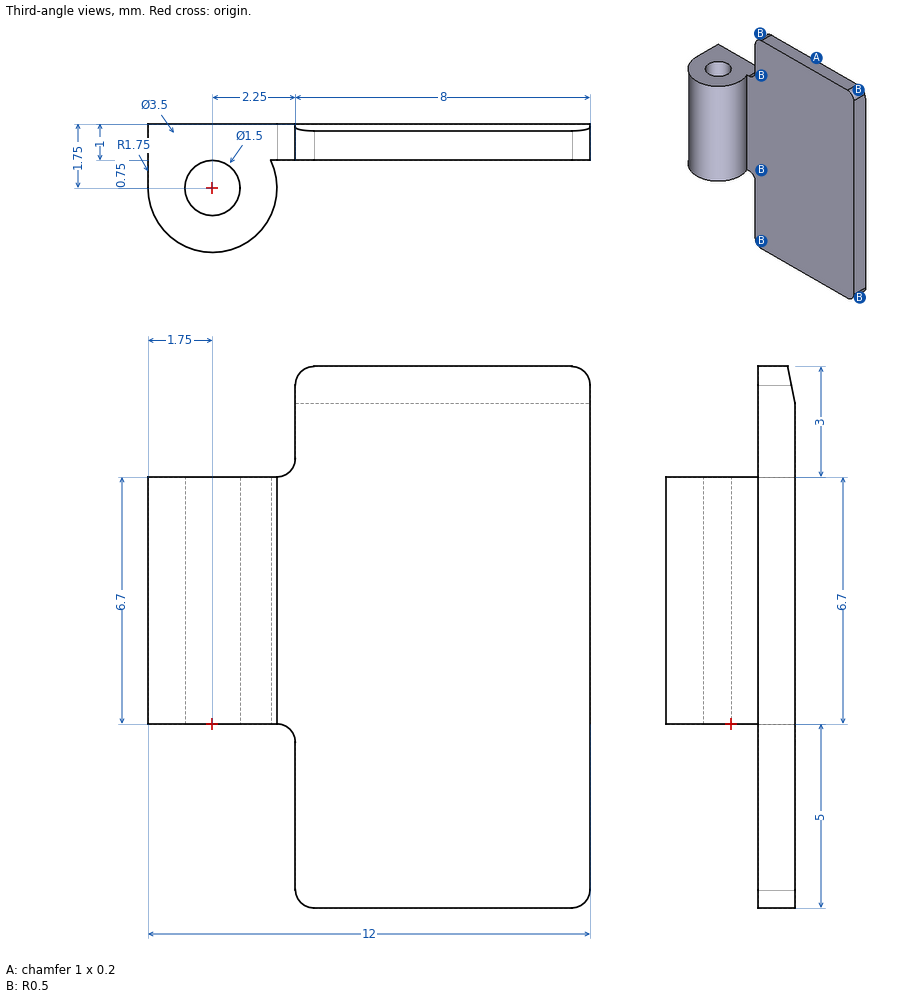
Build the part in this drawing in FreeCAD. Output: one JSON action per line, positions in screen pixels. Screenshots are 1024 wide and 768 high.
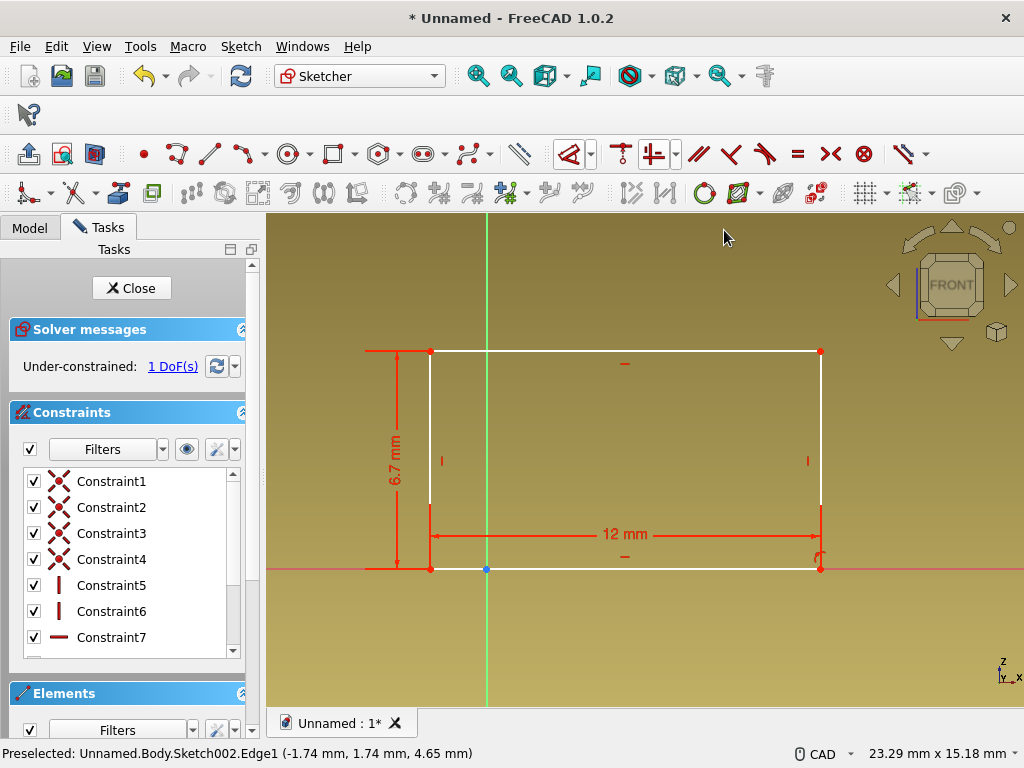
{"action": "left_click", "coordinate": [430, 351]}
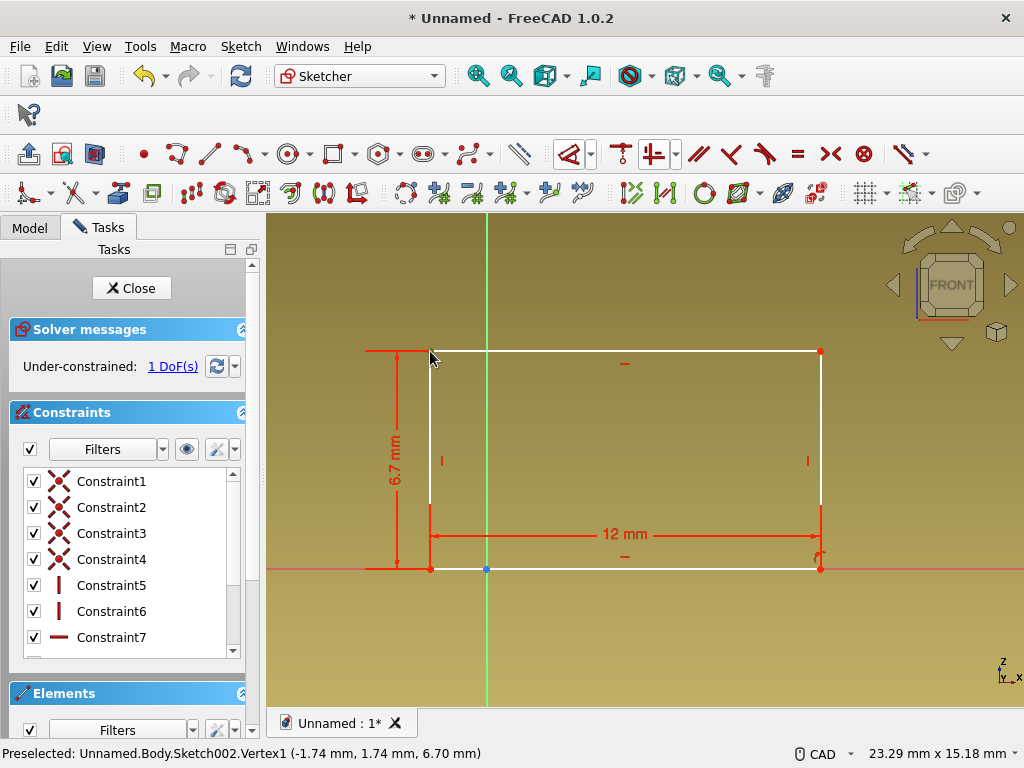
{"action": "left_click", "coordinate": [590, 154]}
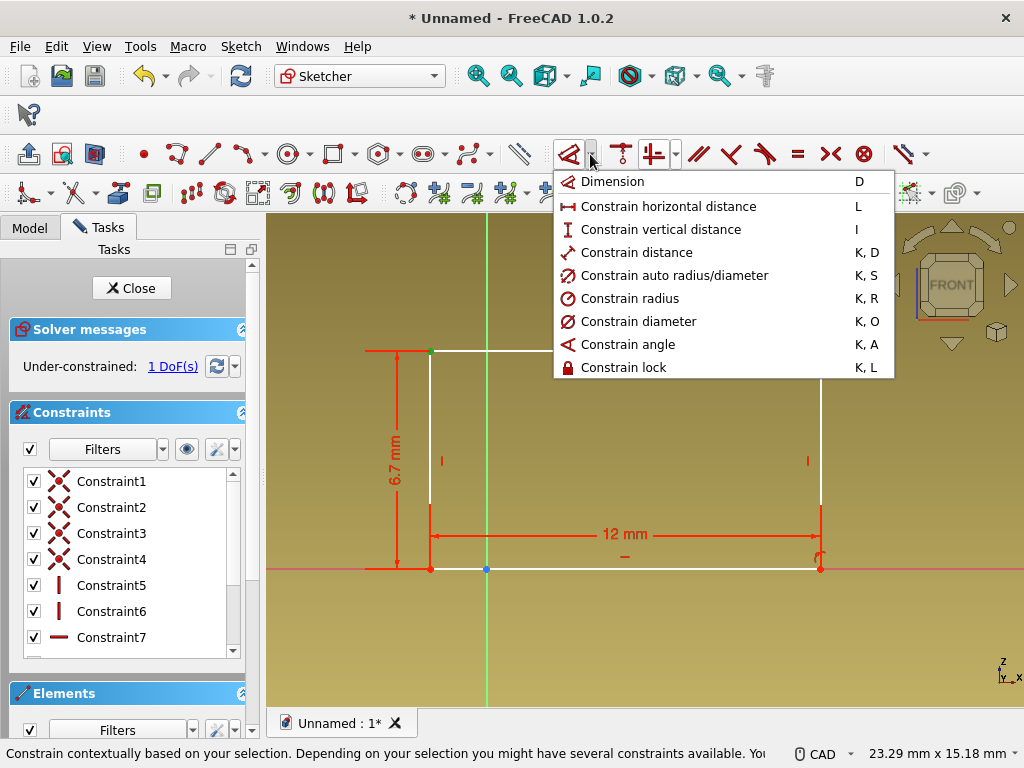
{"action": "left_click", "coordinate": [724, 206]}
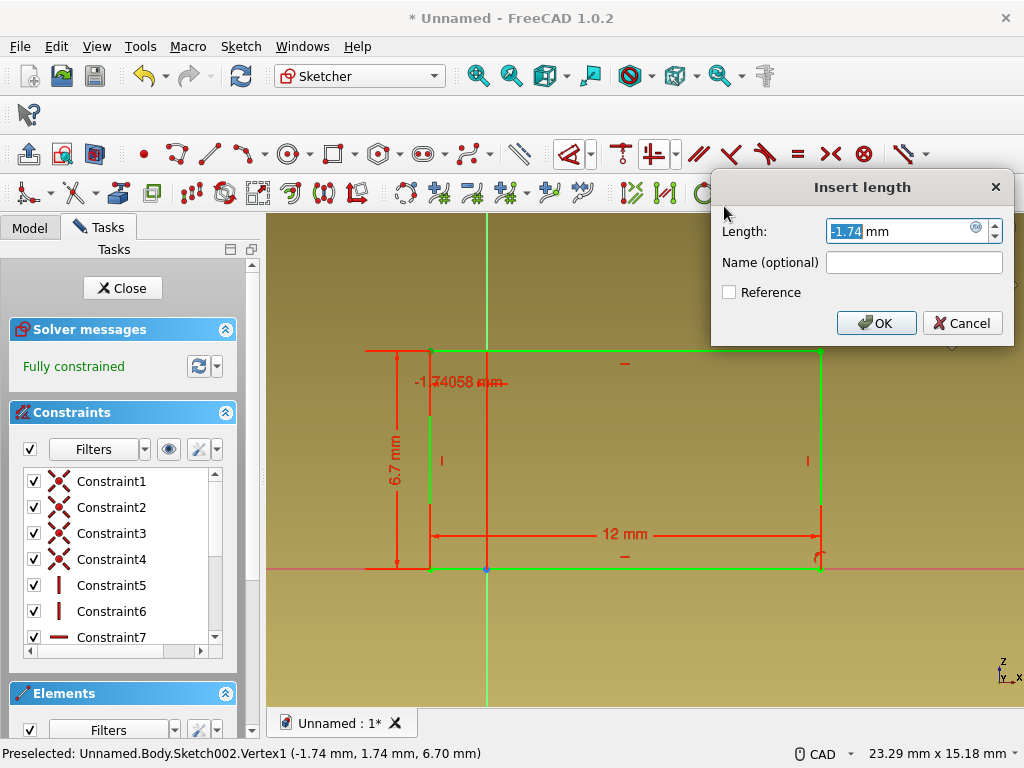
{"action": "type", "text": "-1.75"}
{"action": "key", "text": "Return"}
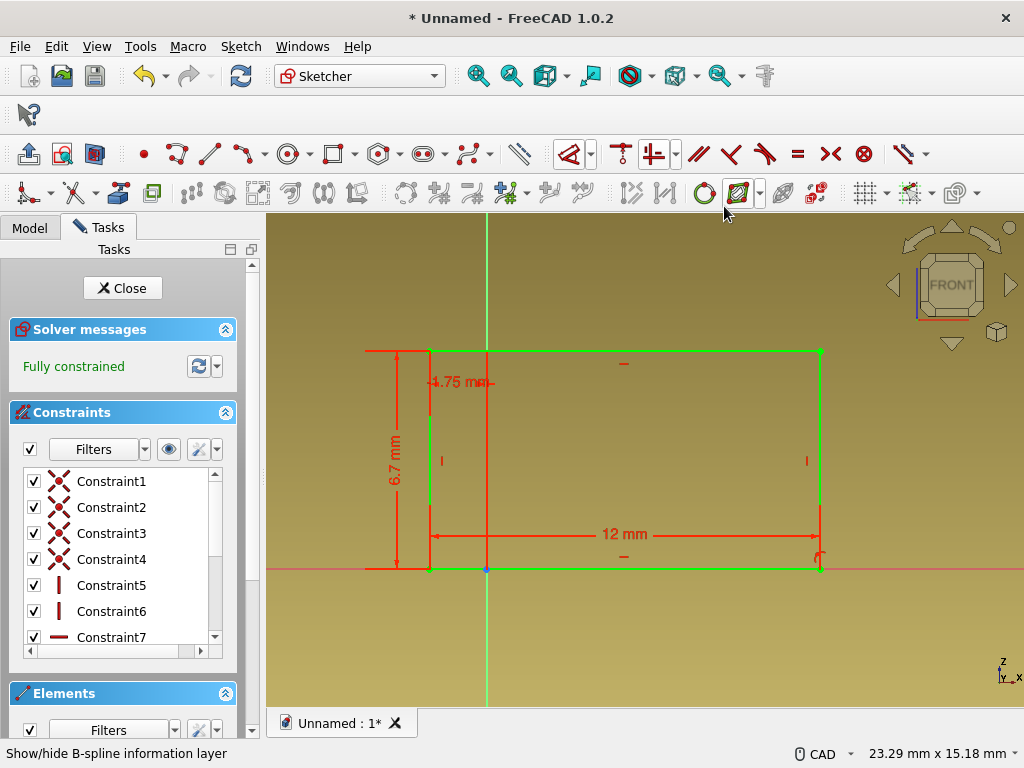
{"action": "left_click", "coordinate": [123, 288]}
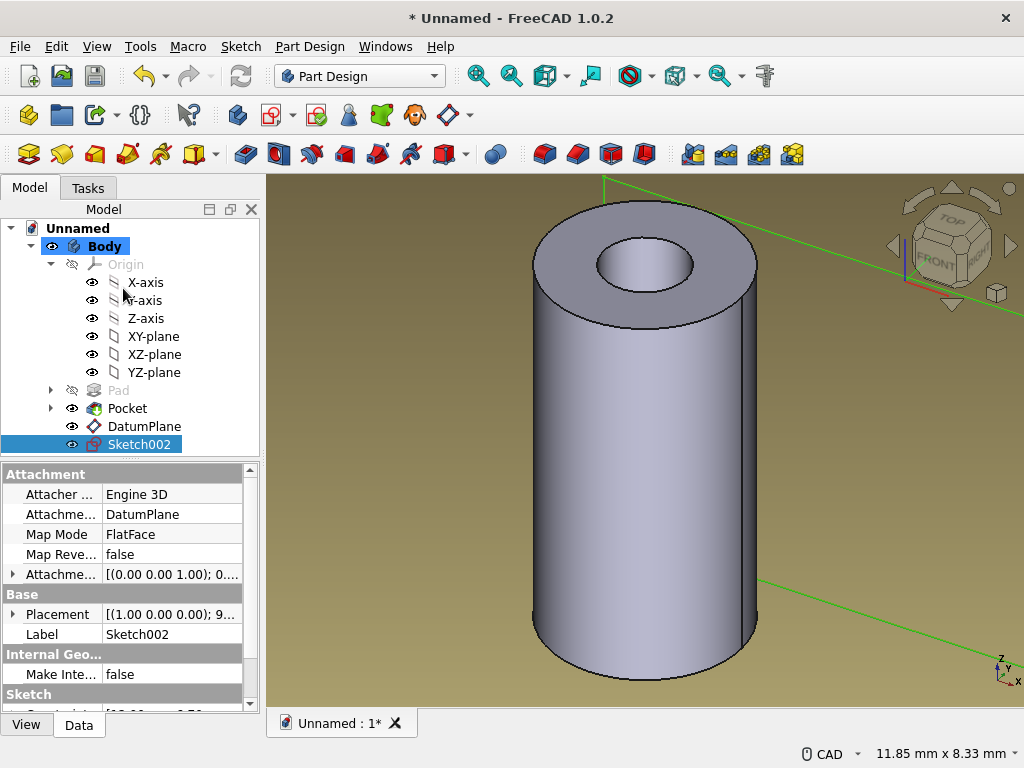
{"action": "left_click", "coordinate": [29, 154]}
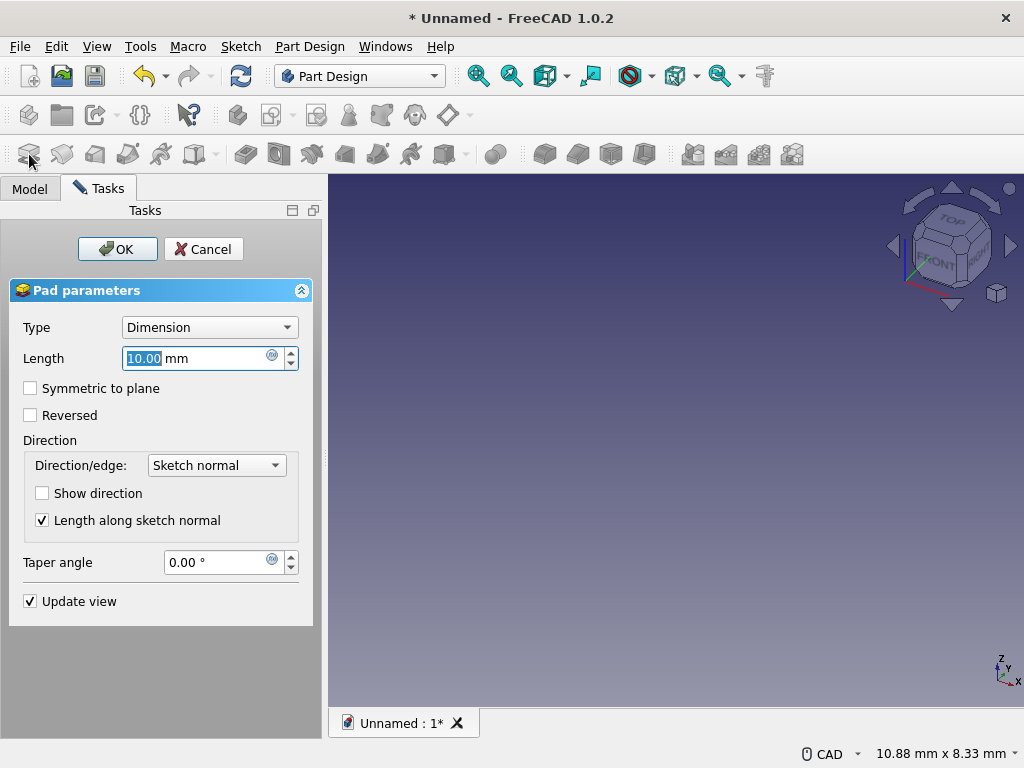
{"action": "type", "text": "1"}
{"action": "key", "text": "Tab"}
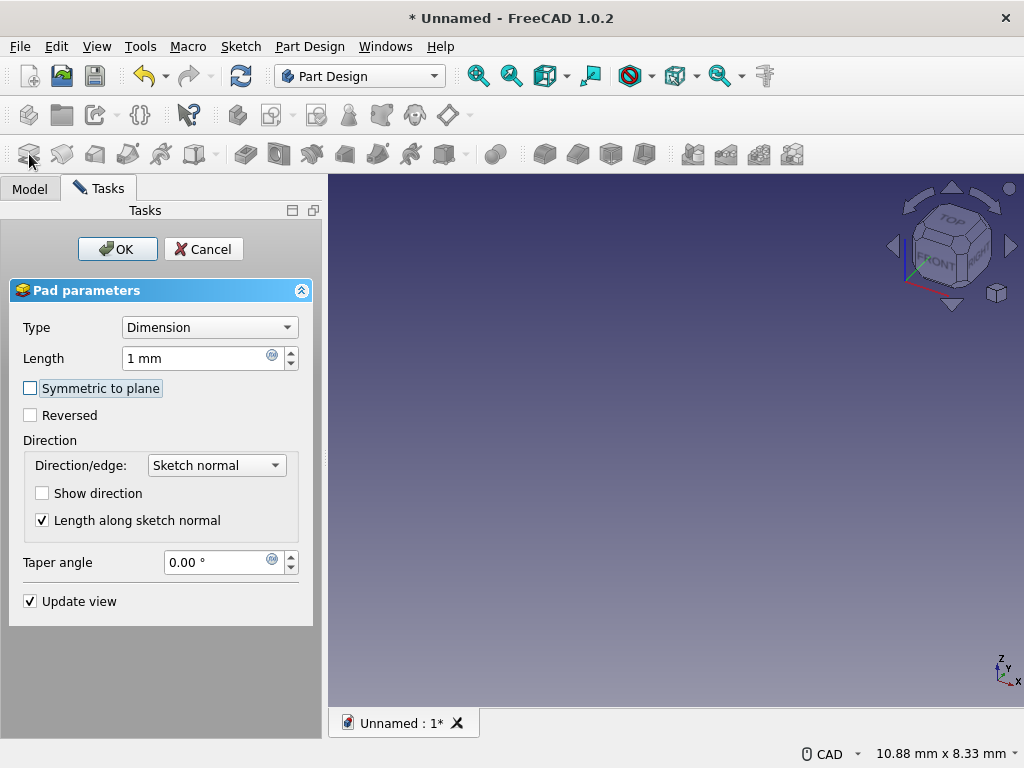
{"action": "left_click", "coordinate": [118, 249]}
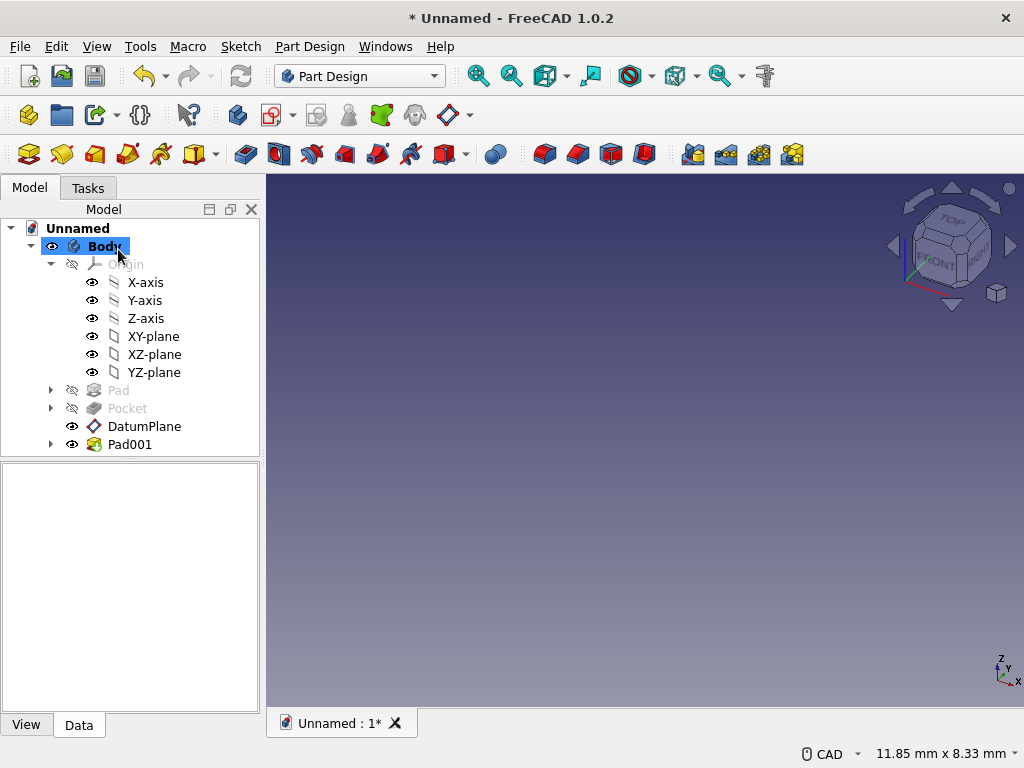
{"action": "left_click", "coordinate": [117, 426]}
{"action": "key", "text": "space"}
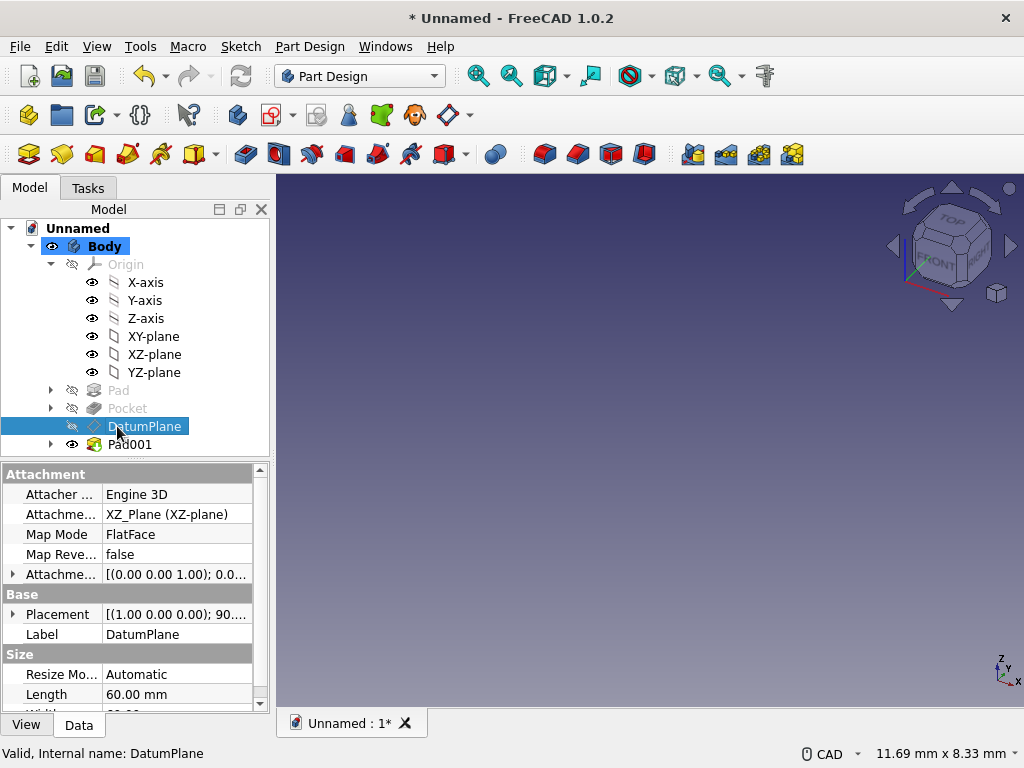
{"action": "left_click", "coordinate": [479, 76]}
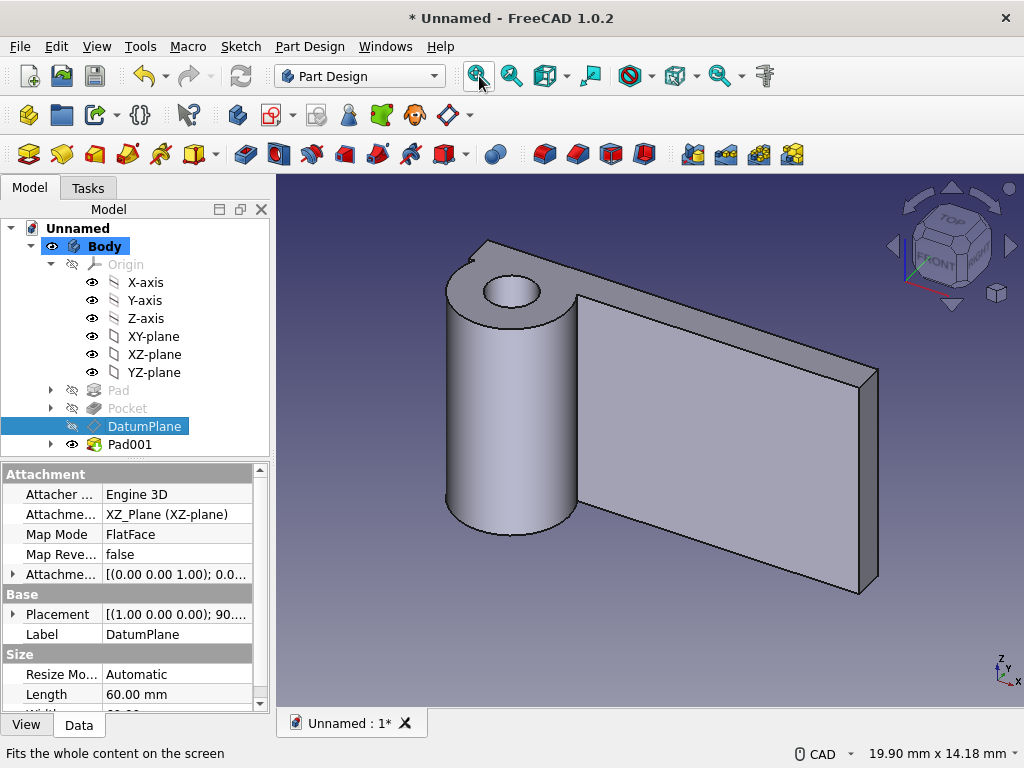
{"action": "key", "text": "5"}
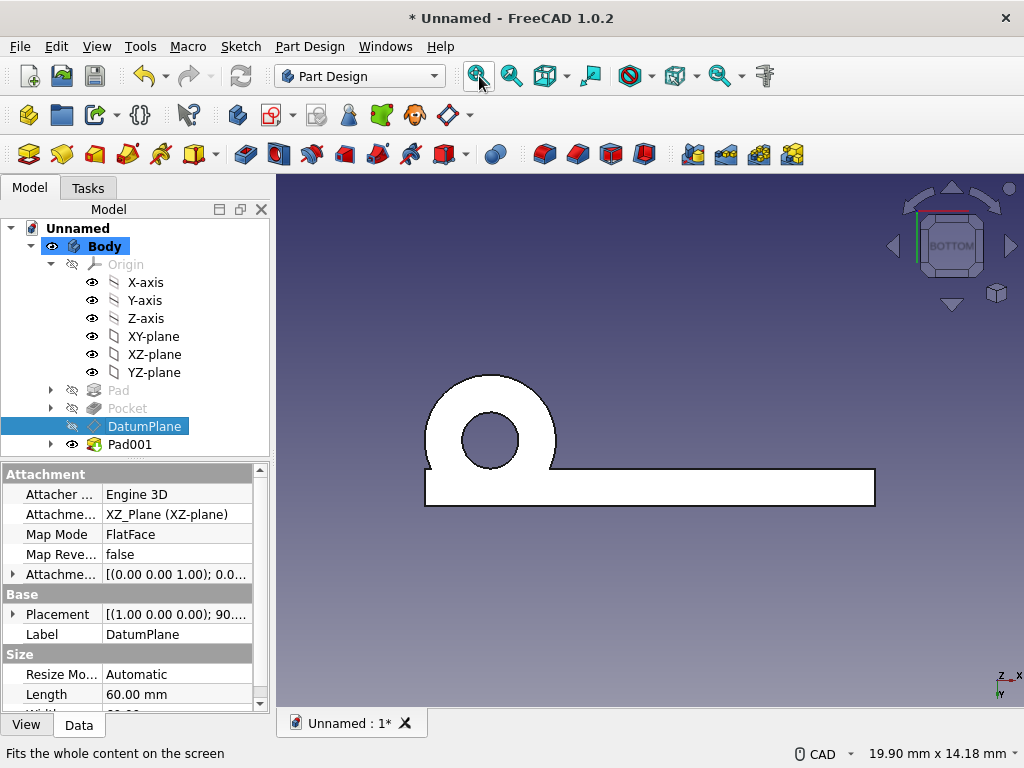
{"action": "left_click", "coordinate": [457, 477]}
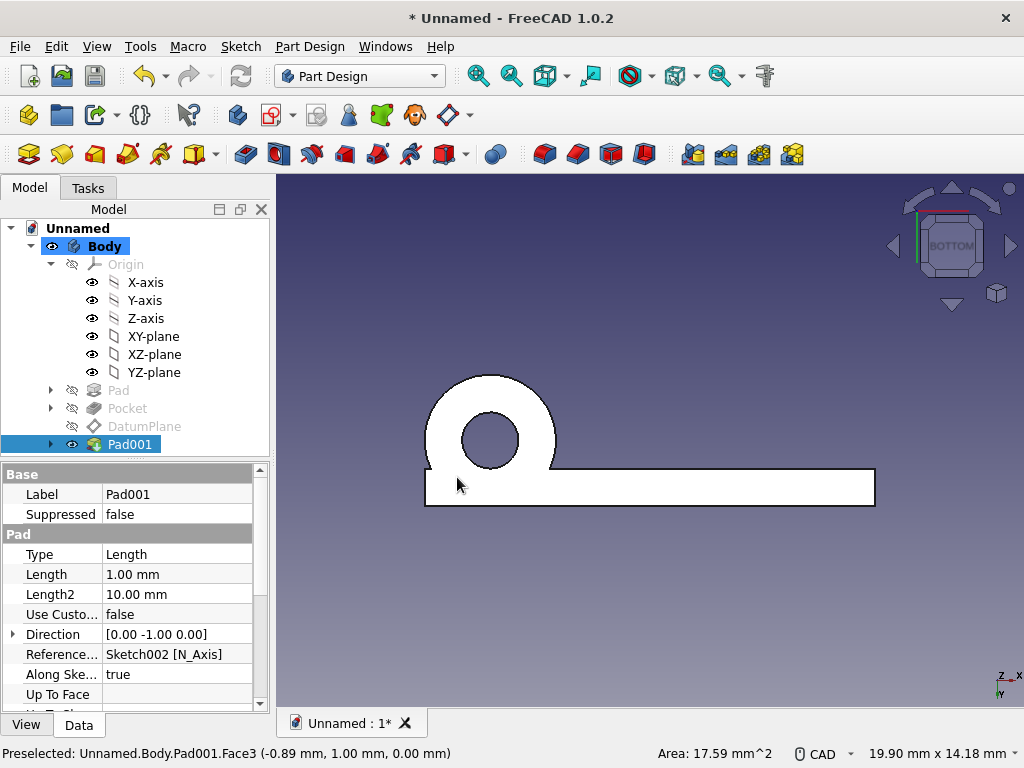
{"action": "left_click", "coordinate": [270, 116]}